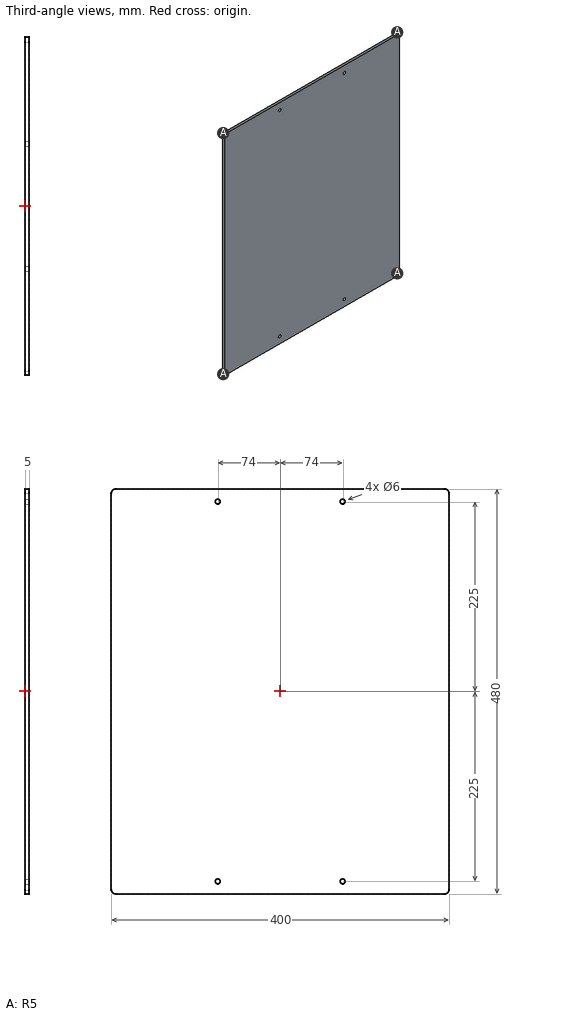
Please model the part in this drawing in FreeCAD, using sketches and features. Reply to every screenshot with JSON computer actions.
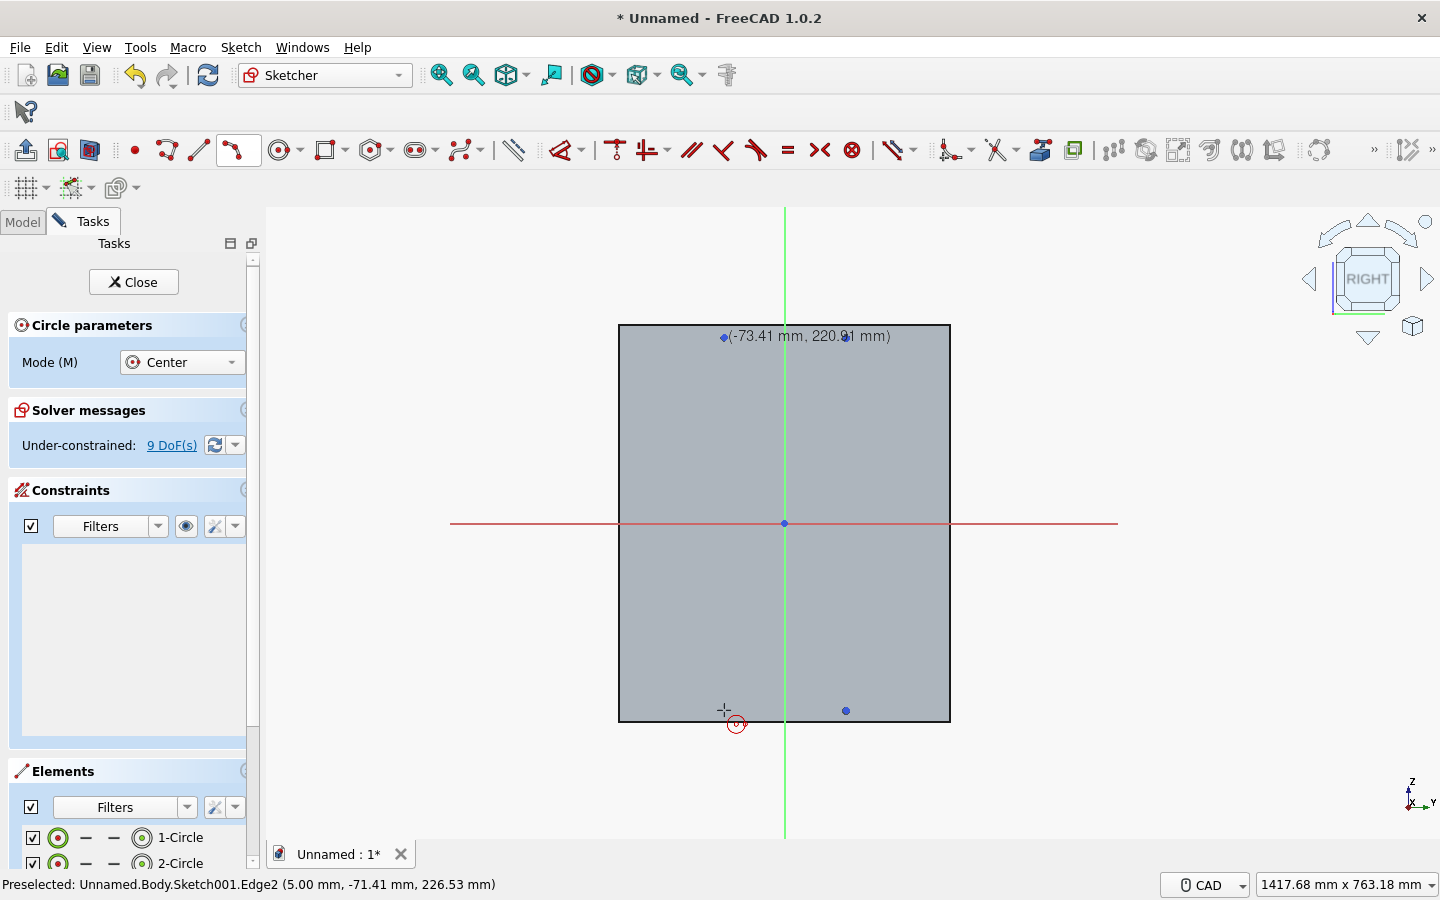
{"action": "left_click", "coordinate": [724, 710]}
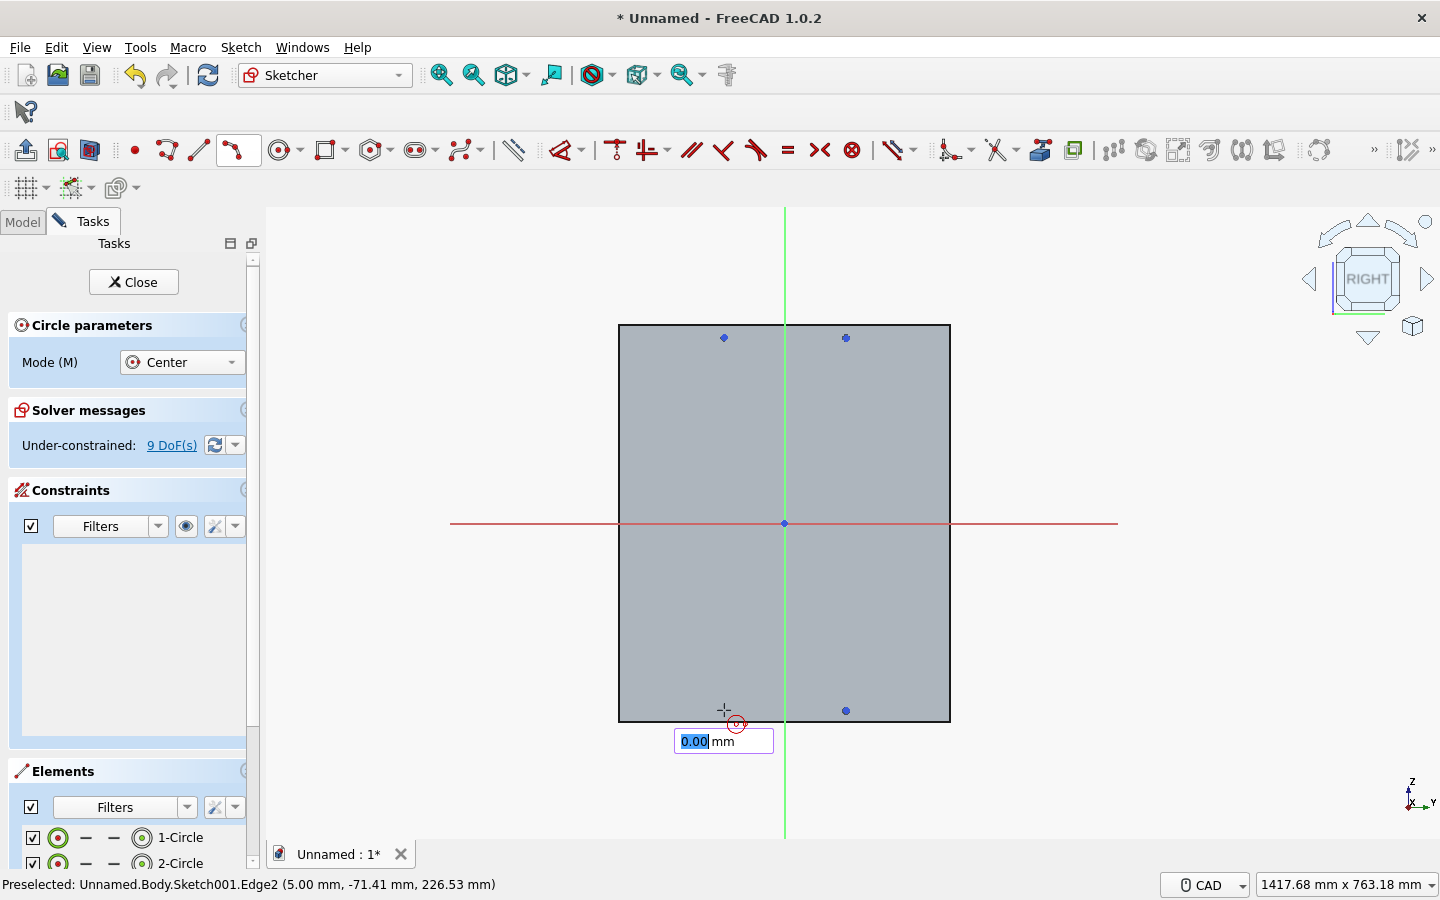
{"action": "scroll", "coordinate": [725, 708], "scroll_direction": "up", "scroll_amount": 10}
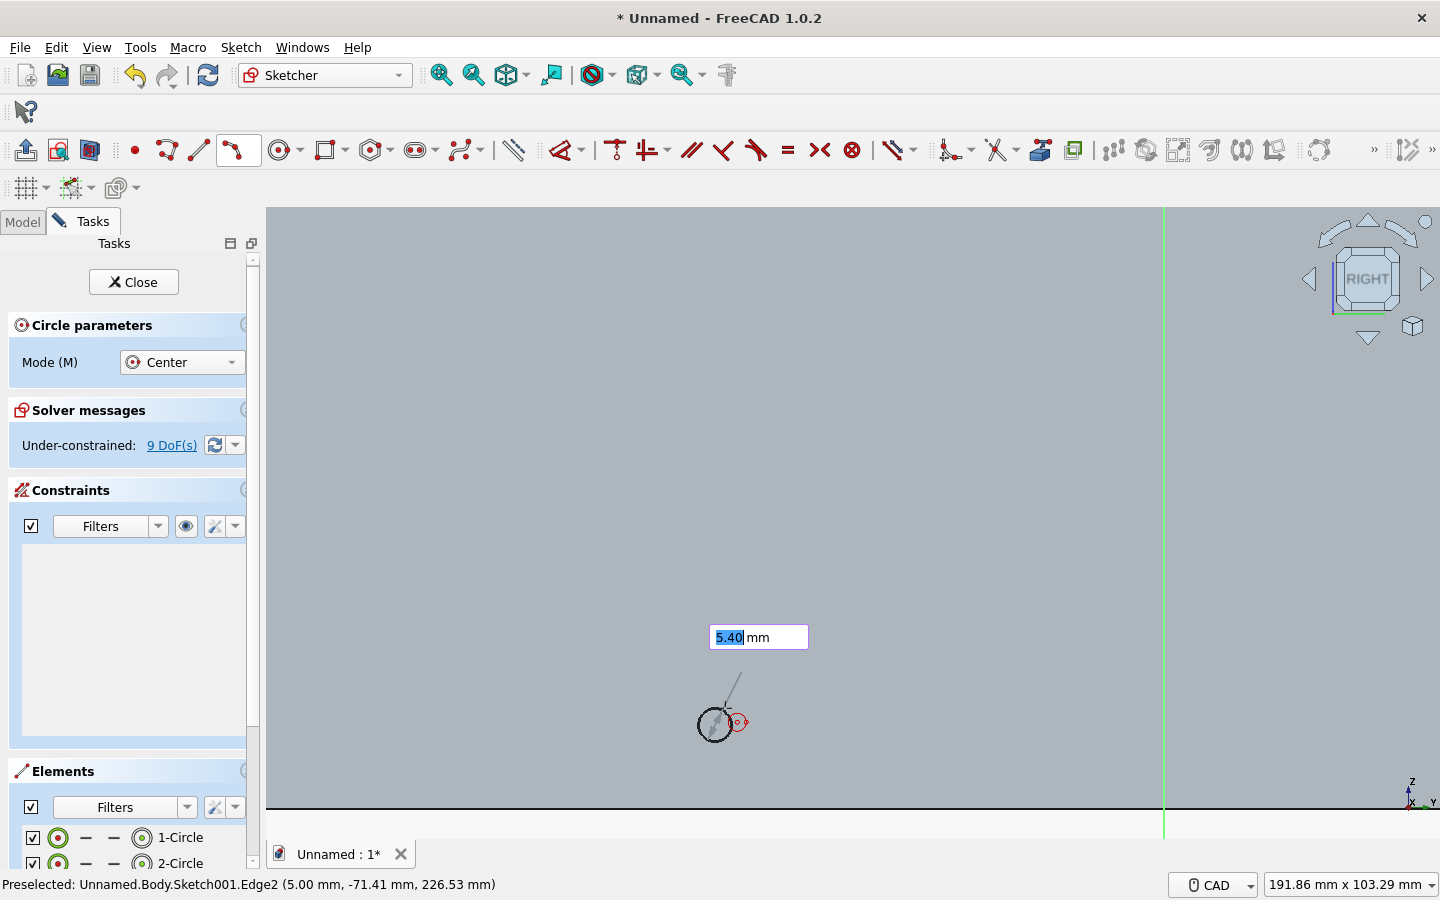
{"action": "left_click", "coordinate": [724, 704]}
{"action": "key", "text": "Escape"}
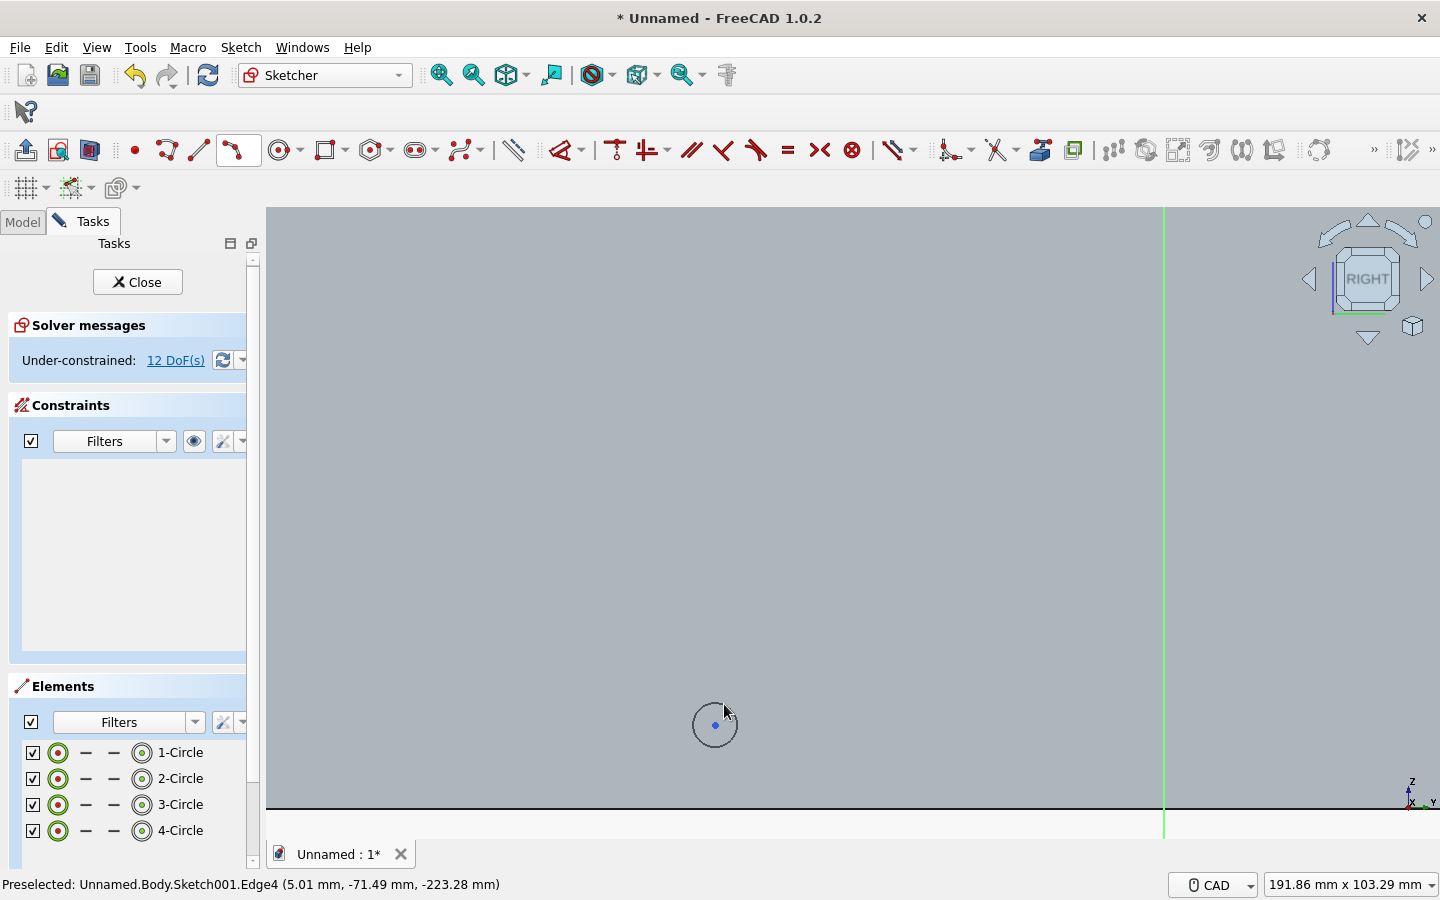
{"action": "scroll", "coordinate": [725, 708], "scroll_direction": "down", "scroll_amount": 10}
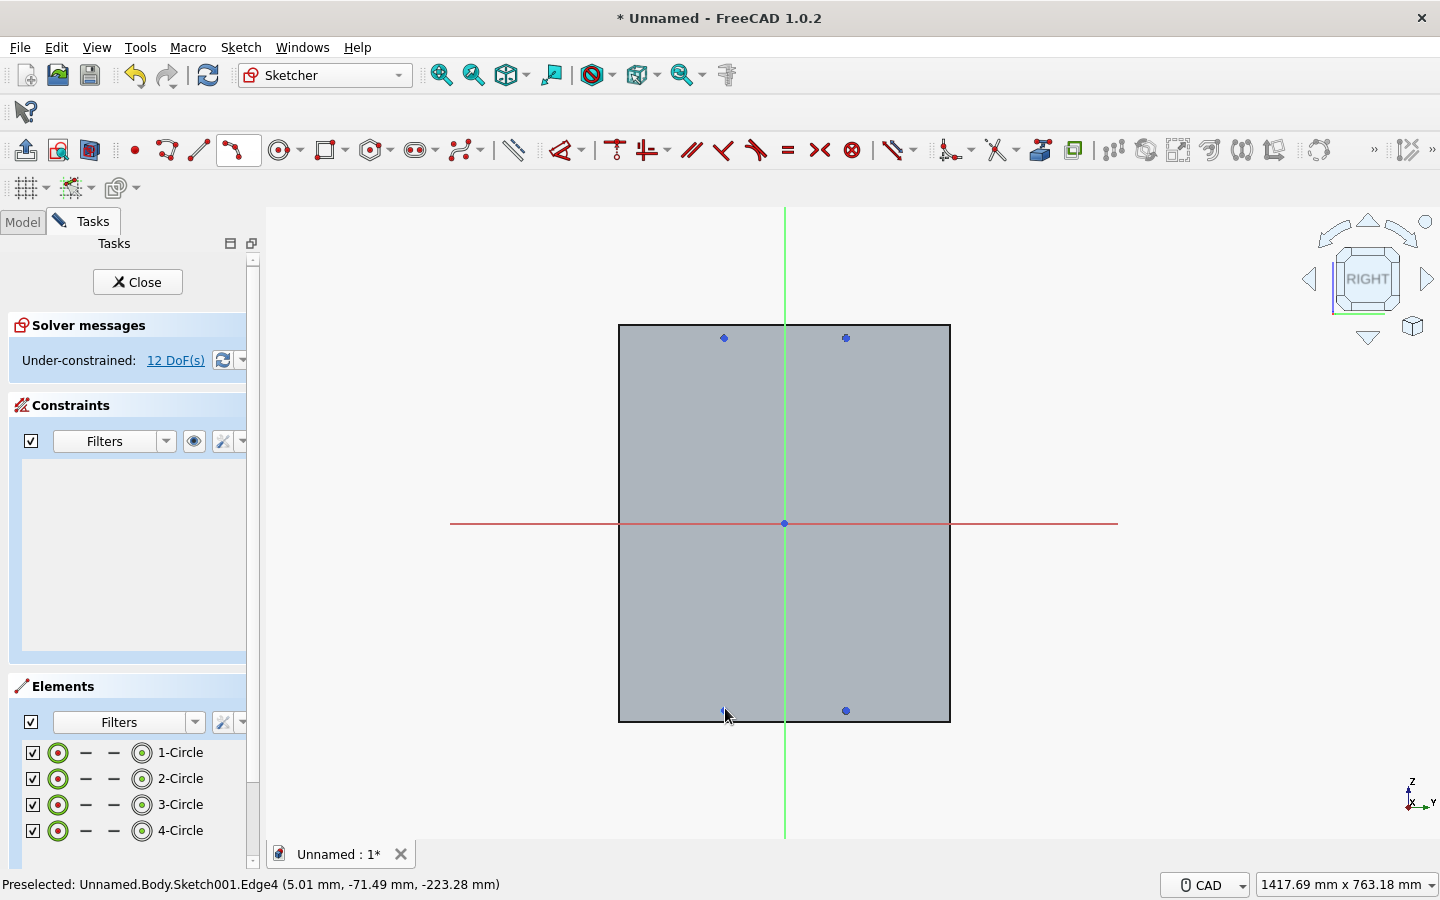
{"action": "scroll", "coordinate": [848, 336], "scroll_direction": "up", "scroll_amount": 8}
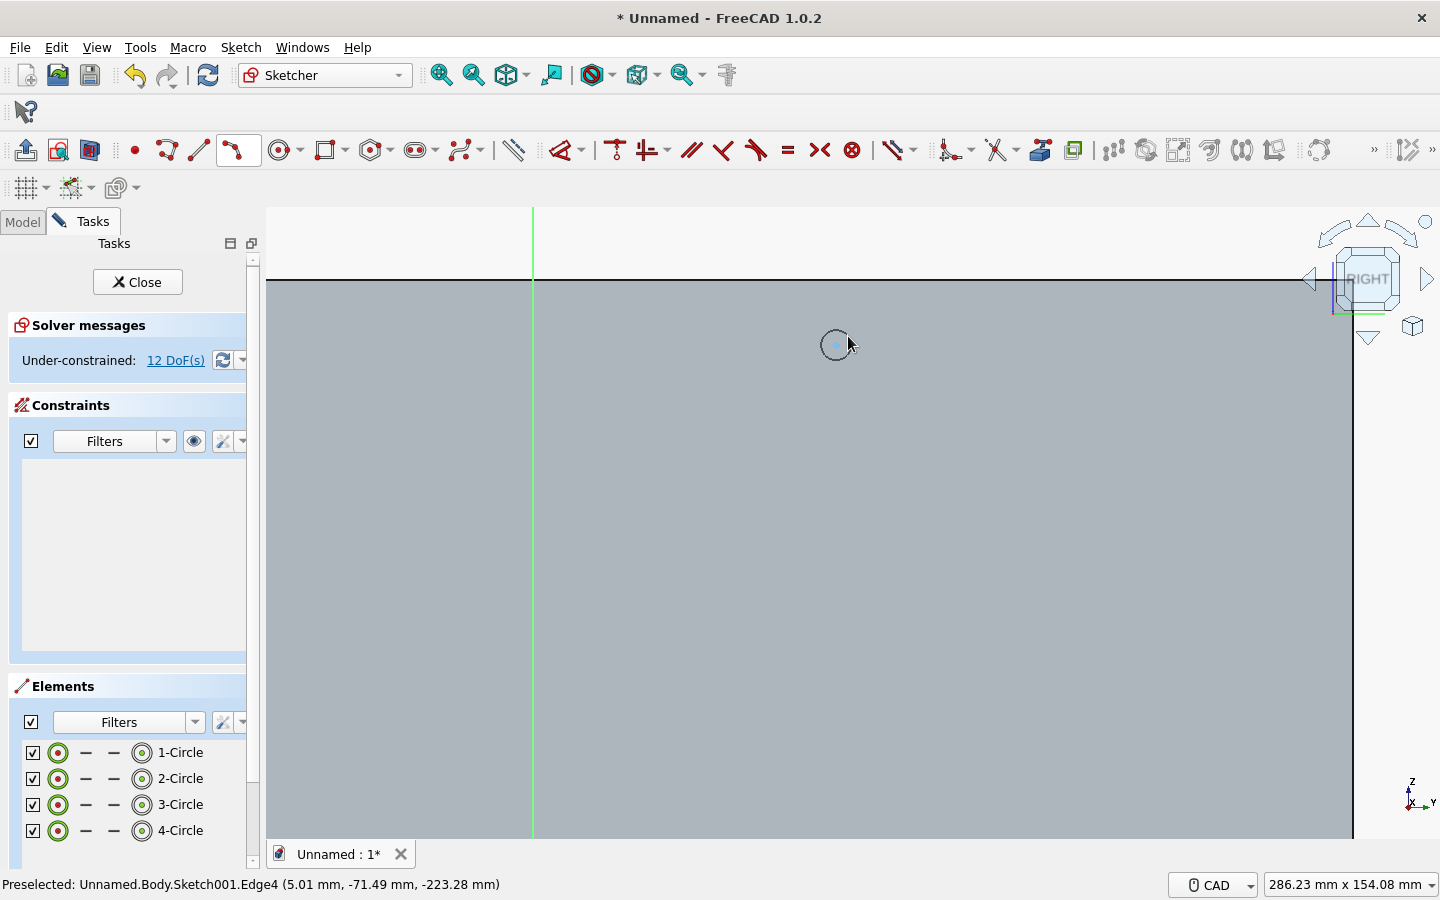
{"action": "left_click", "coordinate": [847, 334]}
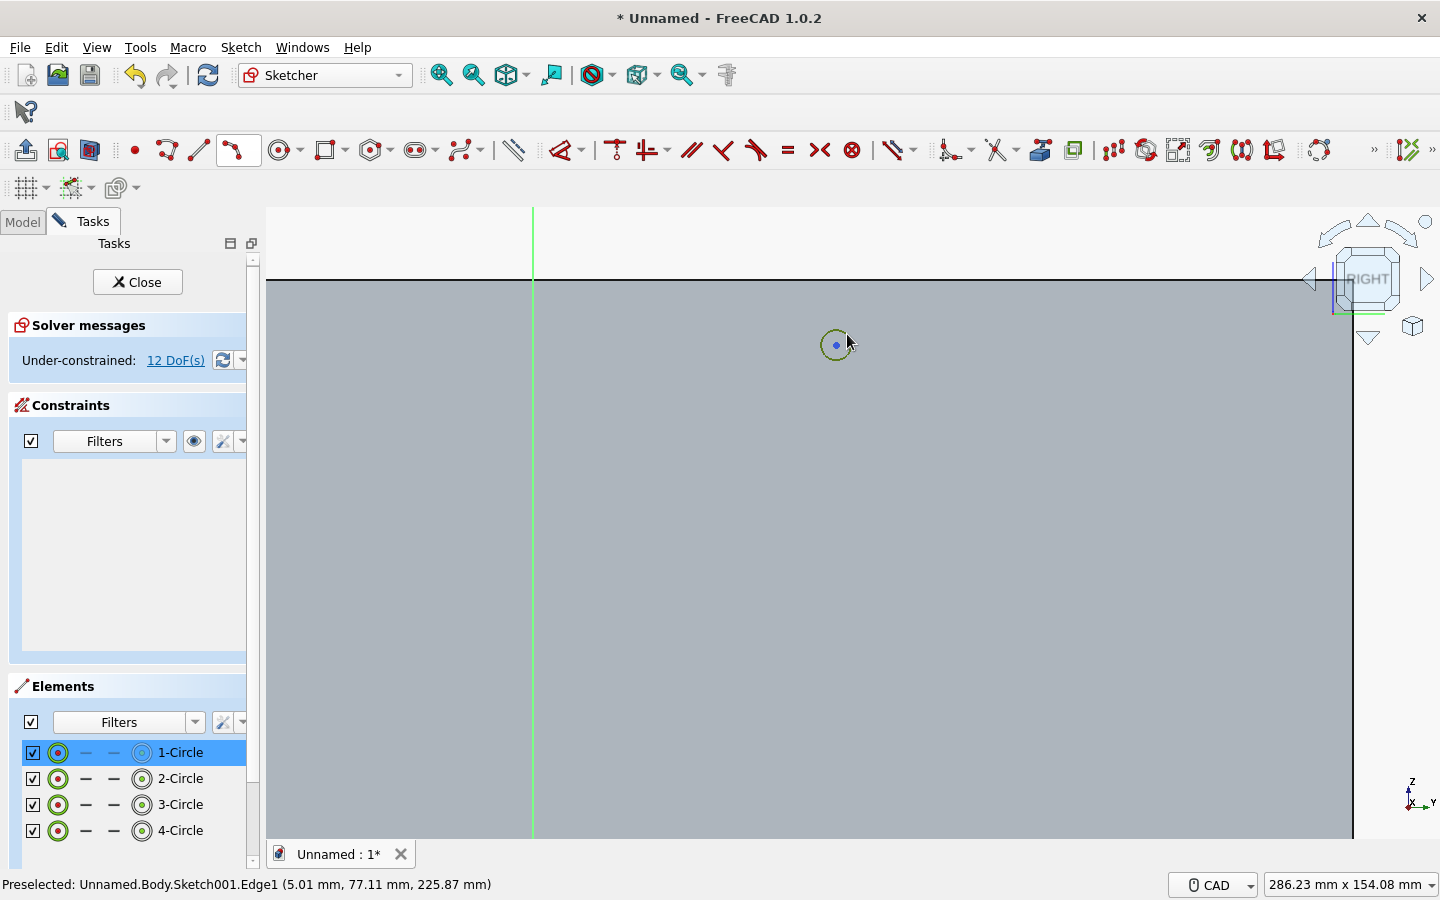
{"action": "scroll", "coordinate": [848, 335], "scroll_direction": "down", "scroll_amount": 8}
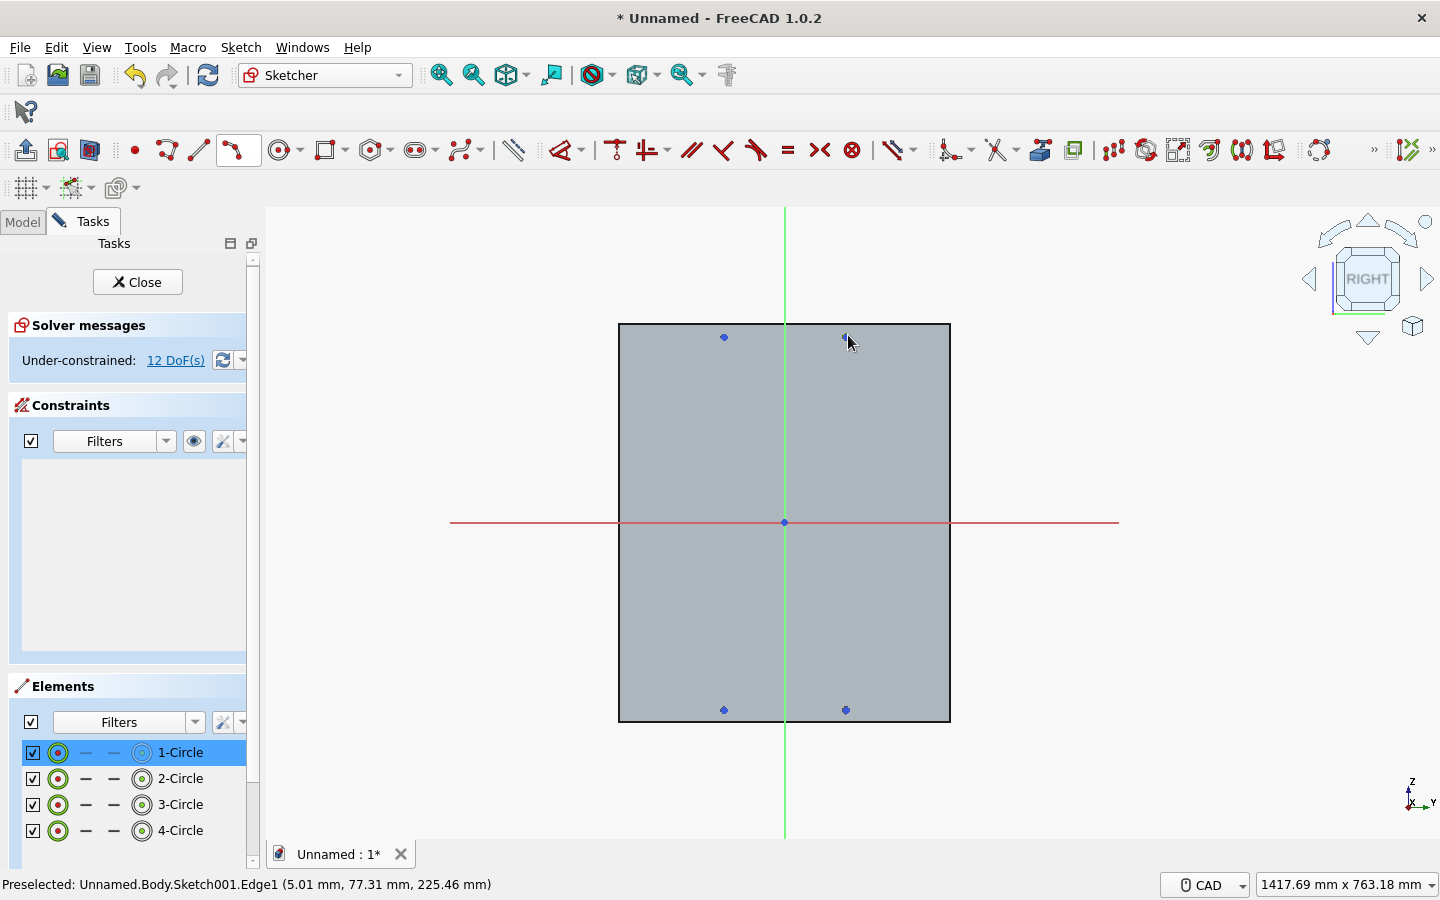
{"action": "scroll", "coordinate": [848, 708], "scroll_direction": "up", "scroll_amount": 8}